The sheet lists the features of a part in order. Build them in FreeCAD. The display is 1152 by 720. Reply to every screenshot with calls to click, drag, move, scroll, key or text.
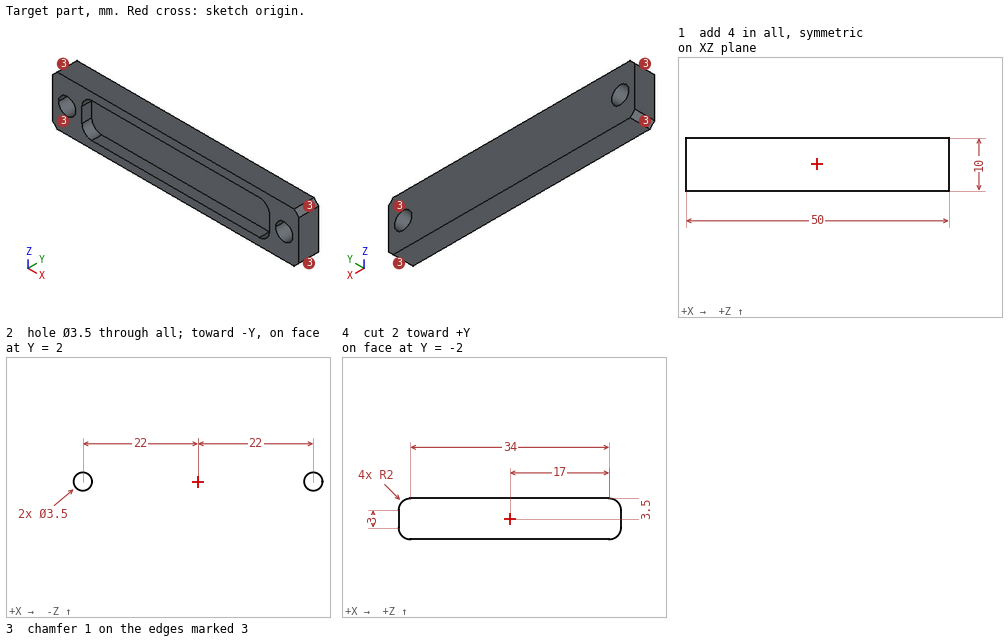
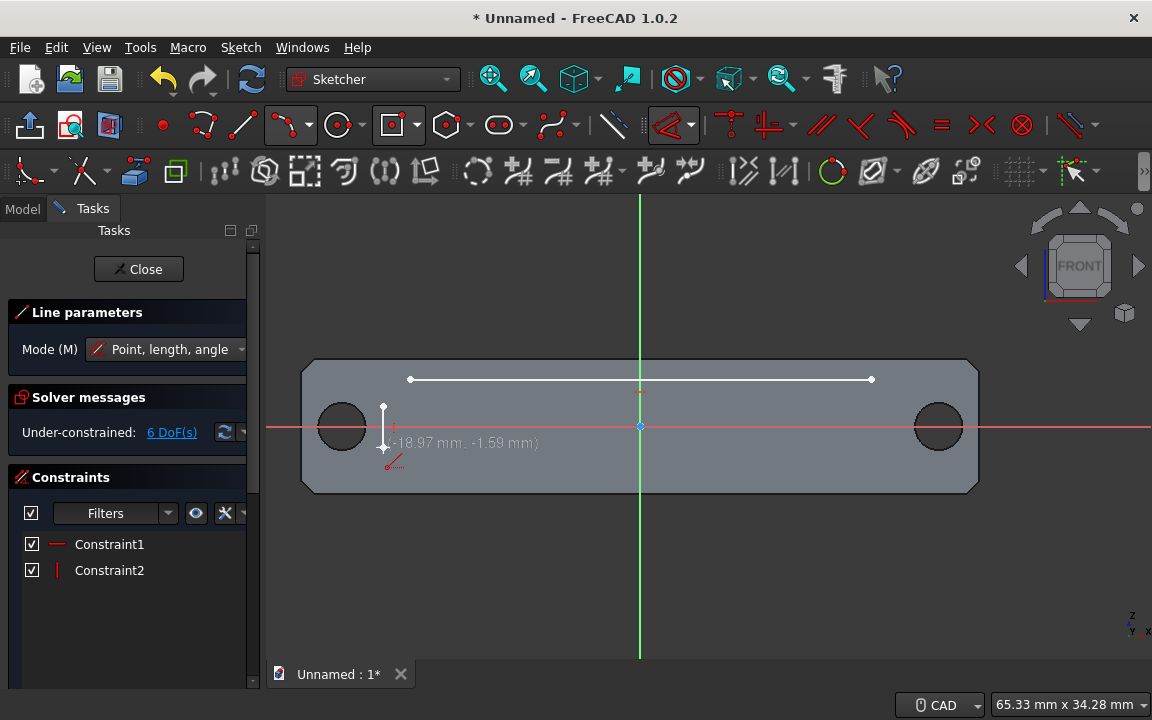
click(410, 474)
click(871, 474)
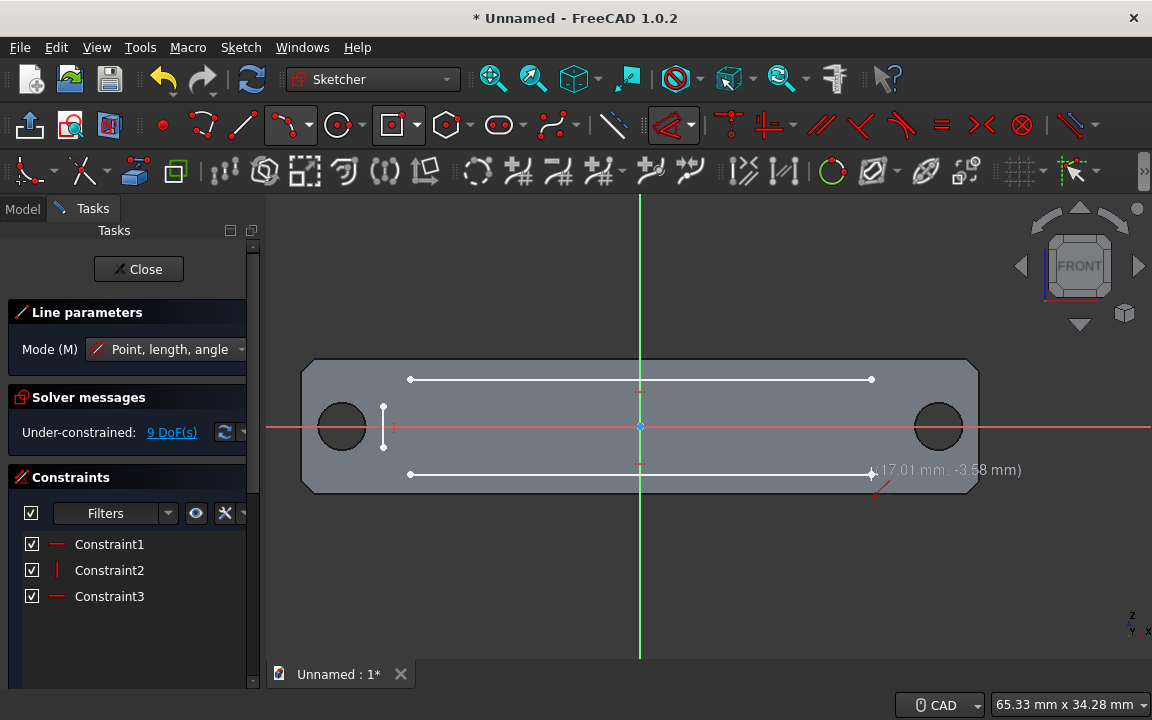
click(898, 447)
click(898, 406)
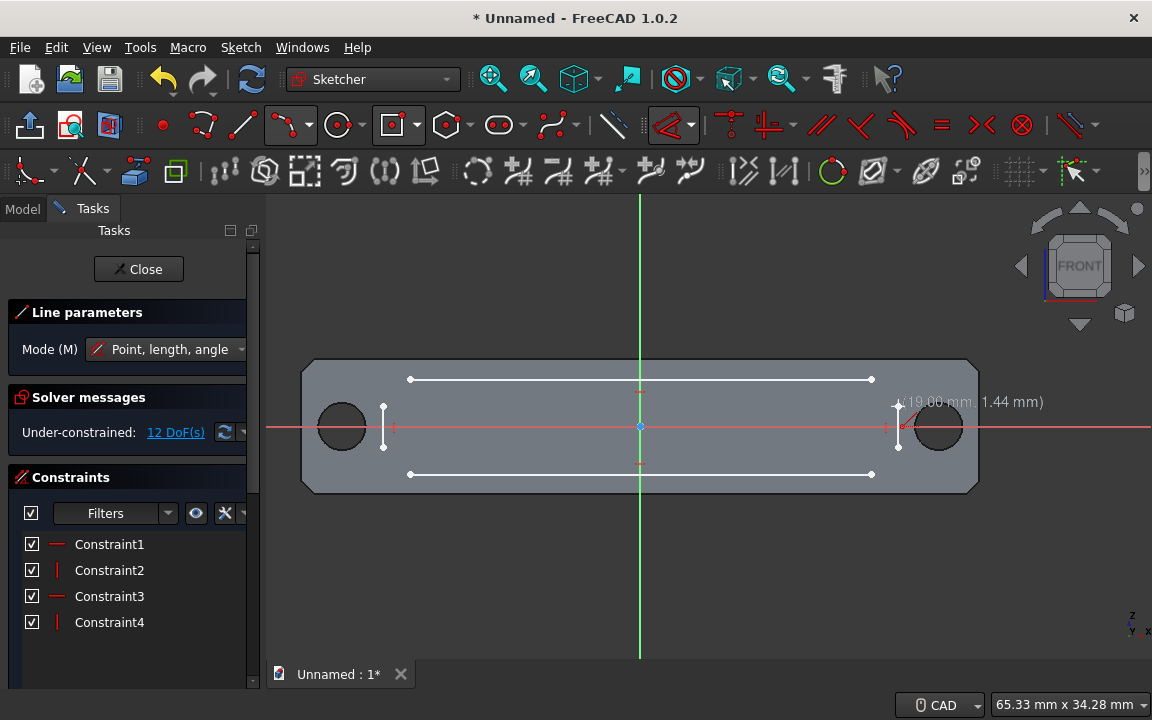
click(284, 126)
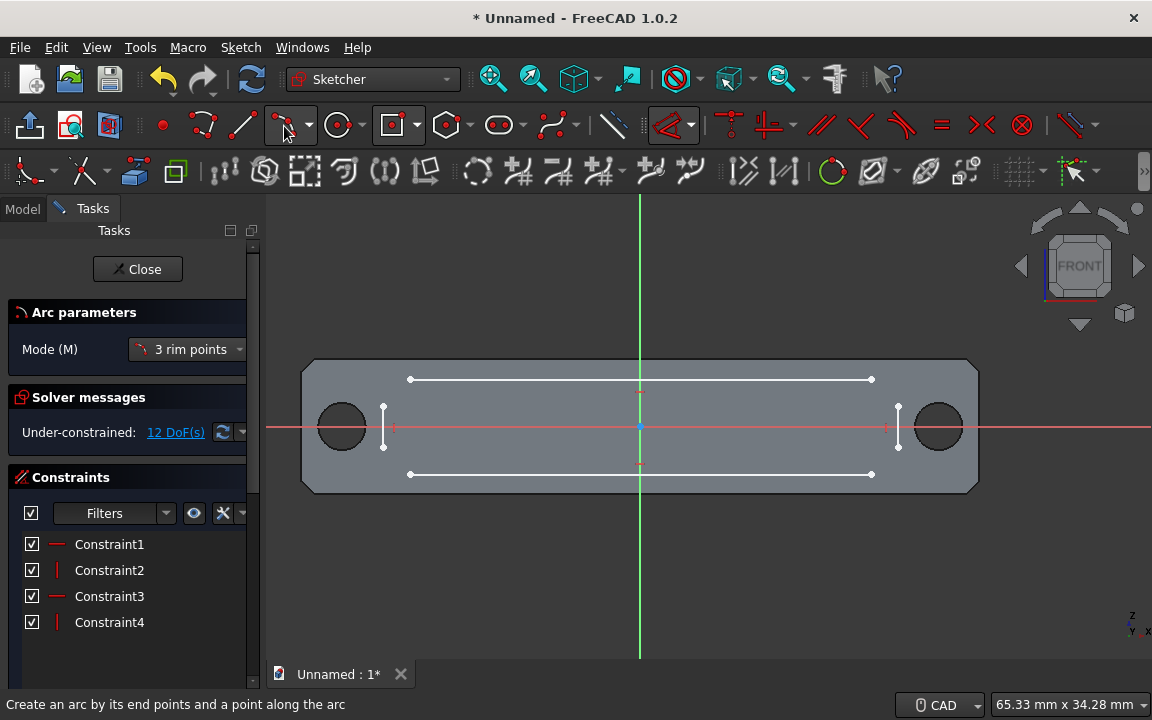
click(410, 380)
click(383, 407)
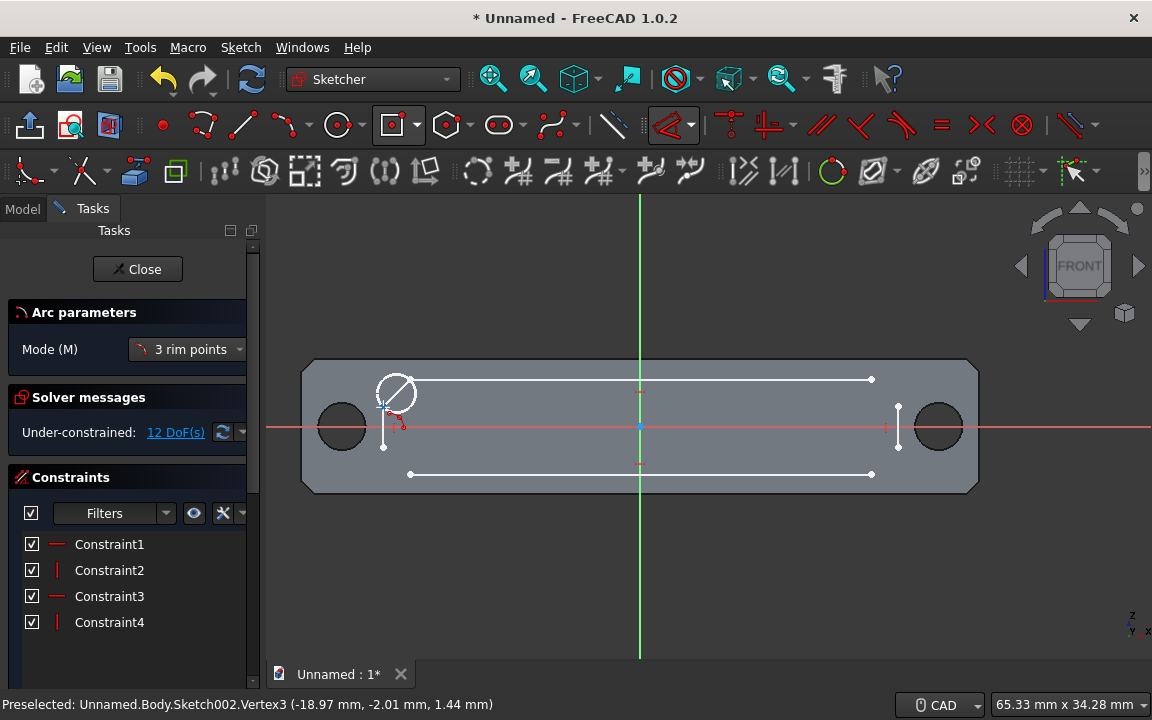
scroll(391, 387, up, 4)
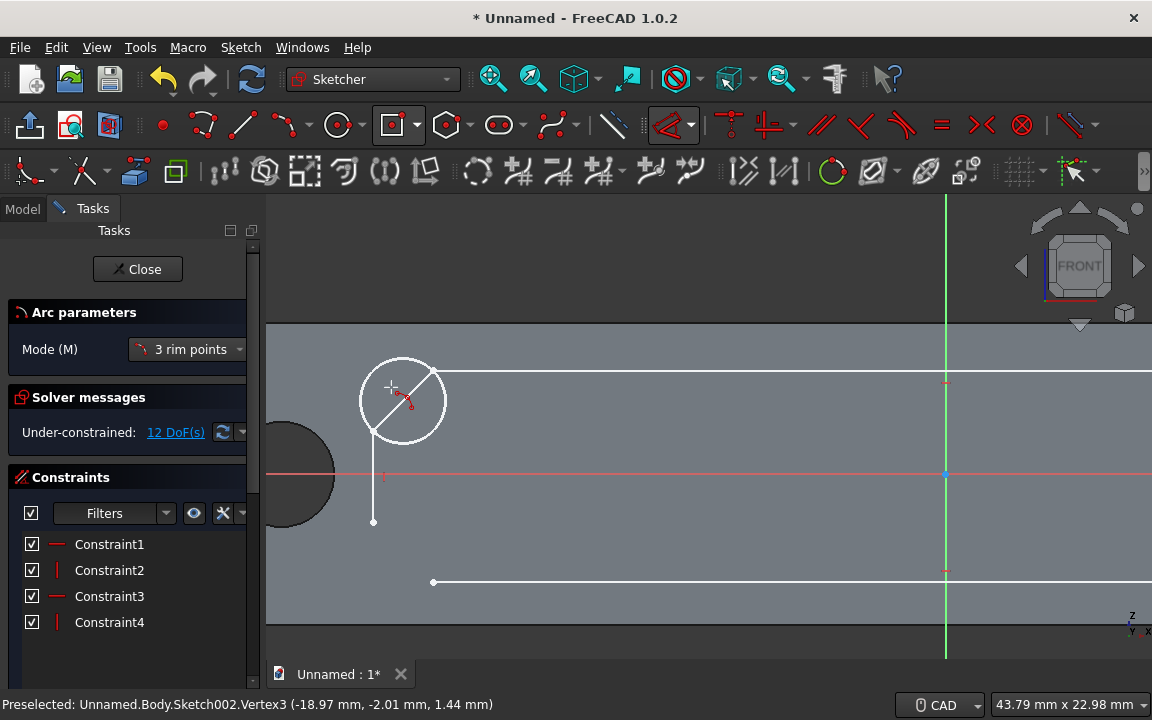
click(390, 386)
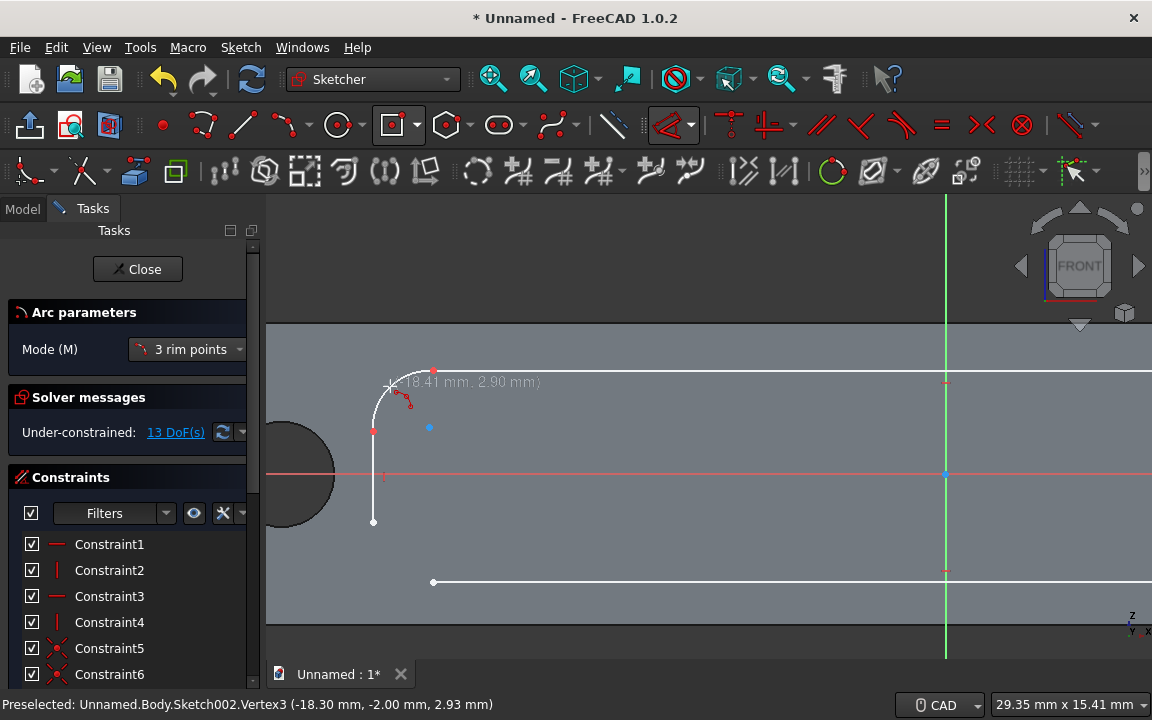
click(373, 522)
click(433, 582)
click(390, 562)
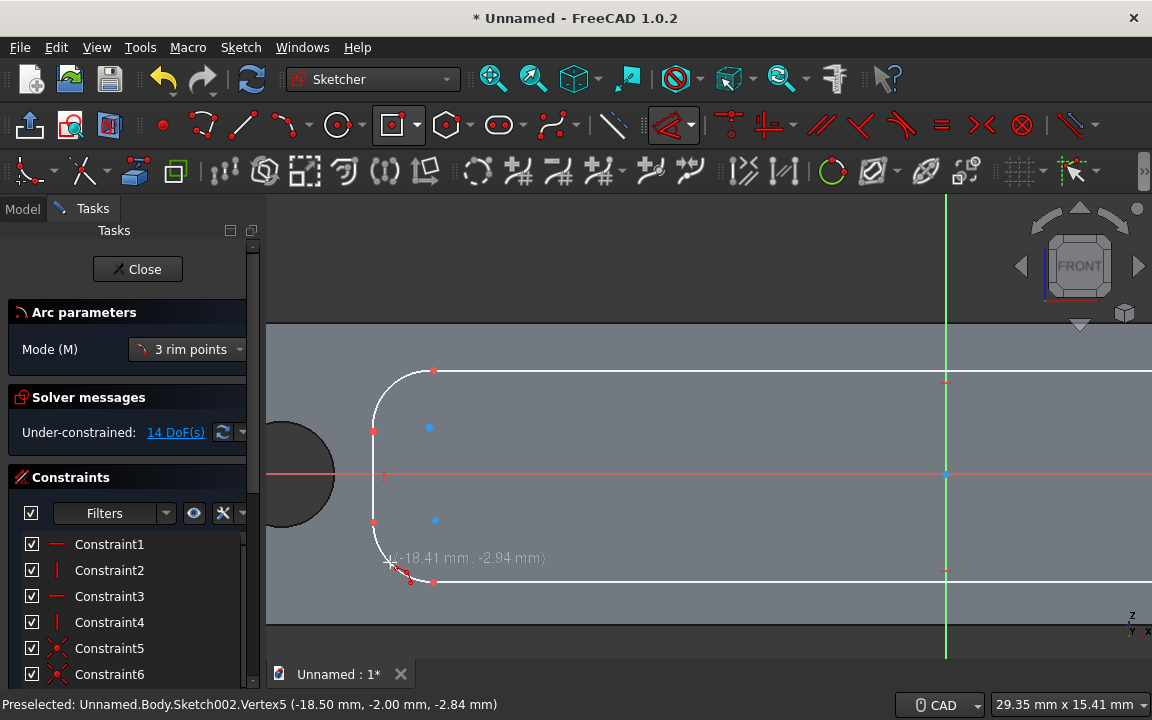
scroll(391, 387, down, 4)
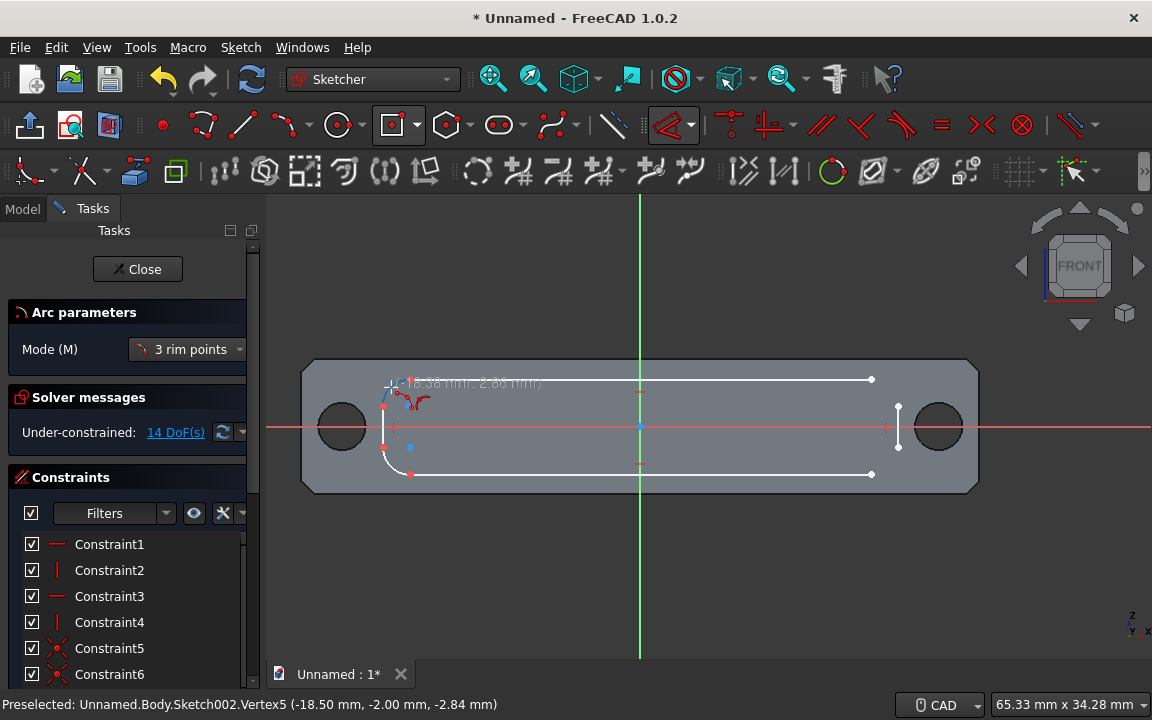
click(871, 475)
click(898, 448)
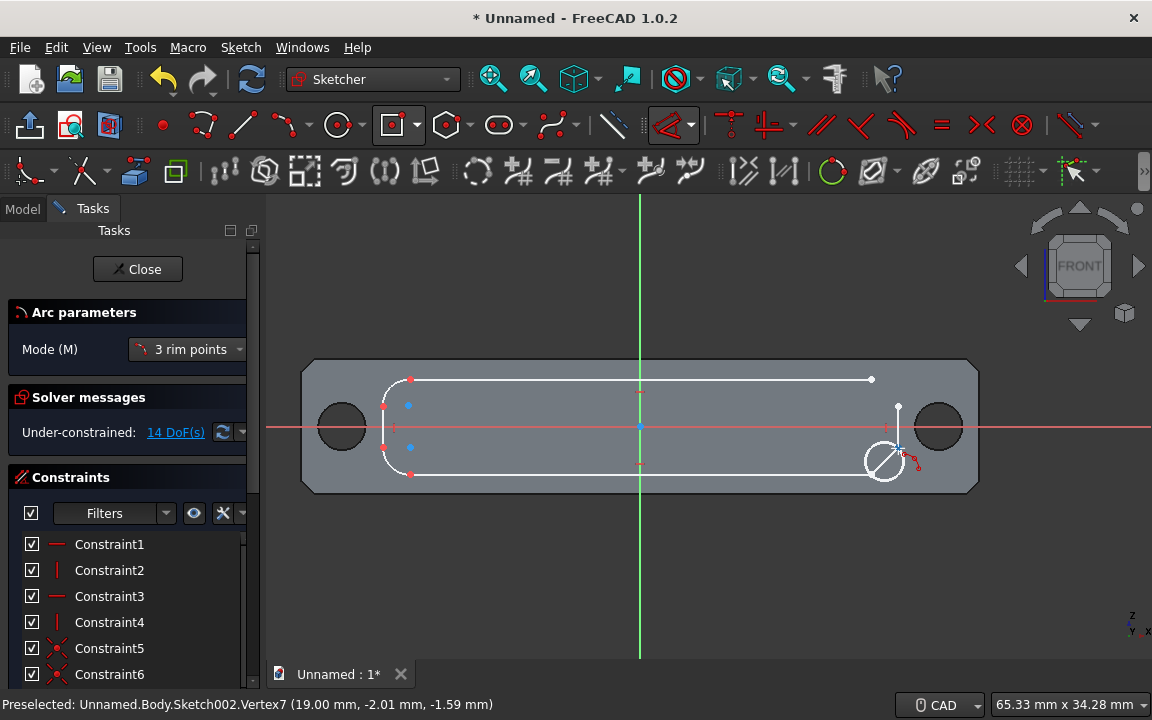
scroll(890, 466, up, 4)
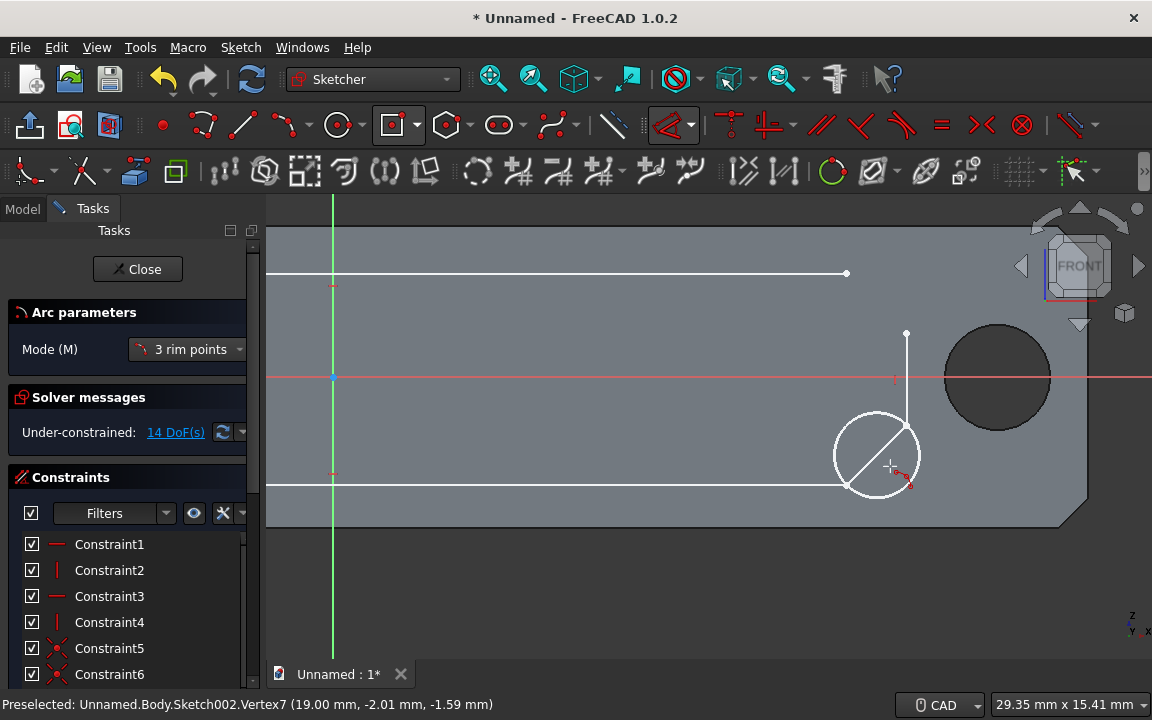
click(889, 465)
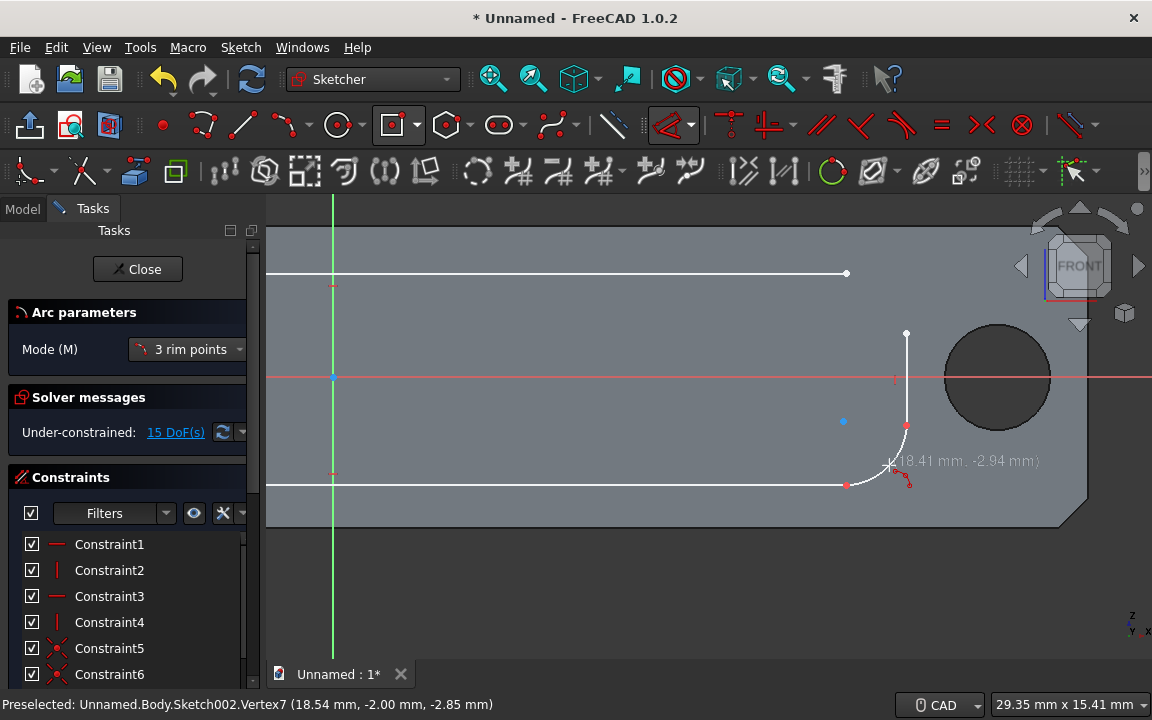
click(907, 334)
click(847, 274)
click(889, 289)
key(Escape)